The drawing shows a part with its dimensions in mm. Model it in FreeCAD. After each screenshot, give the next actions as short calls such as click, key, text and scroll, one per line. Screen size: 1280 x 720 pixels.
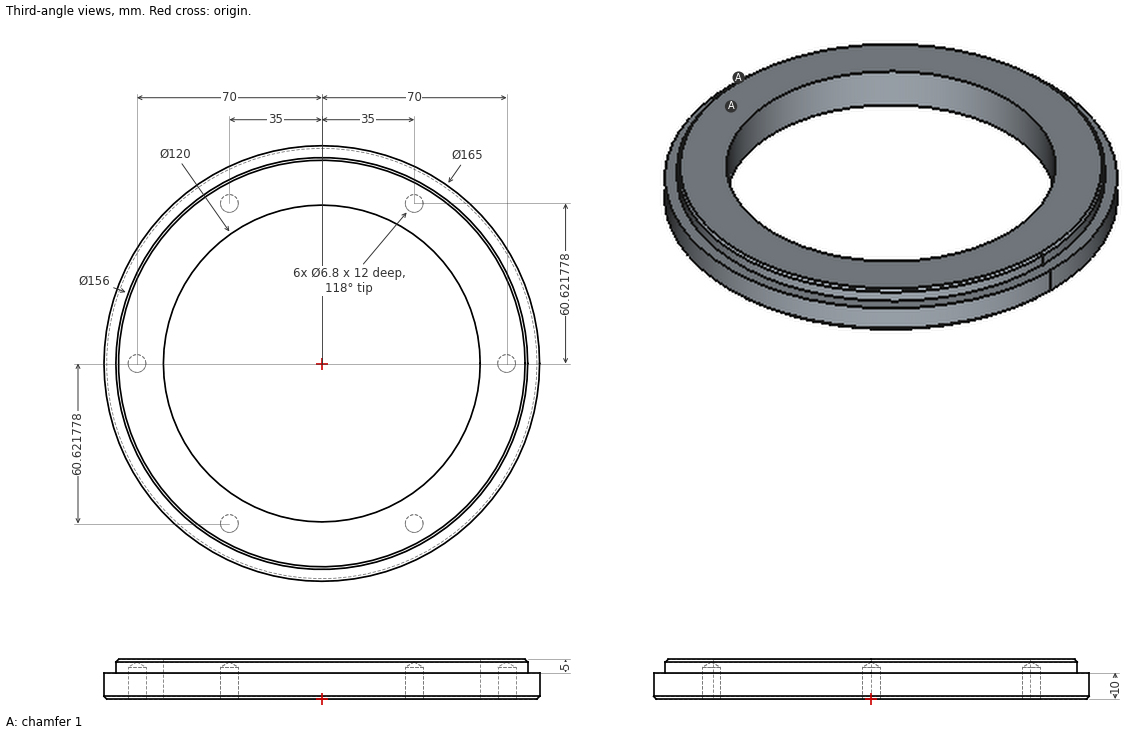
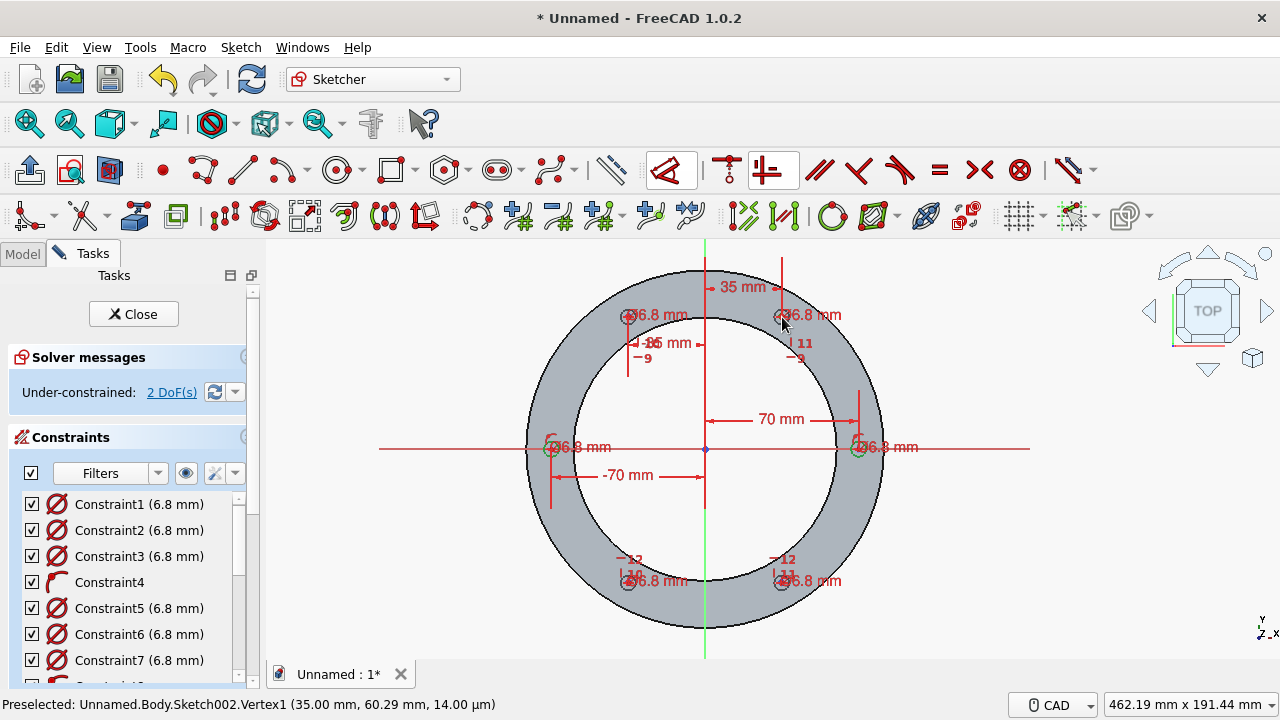
click(692, 170)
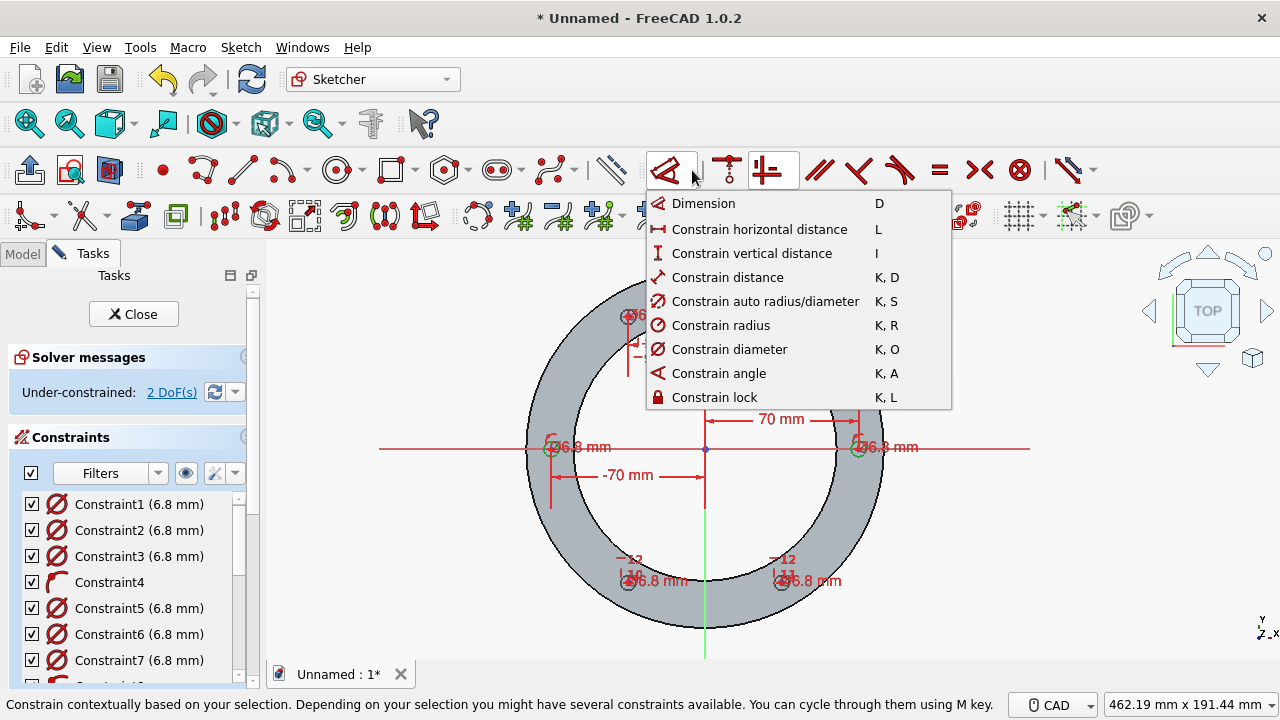
click(799, 253)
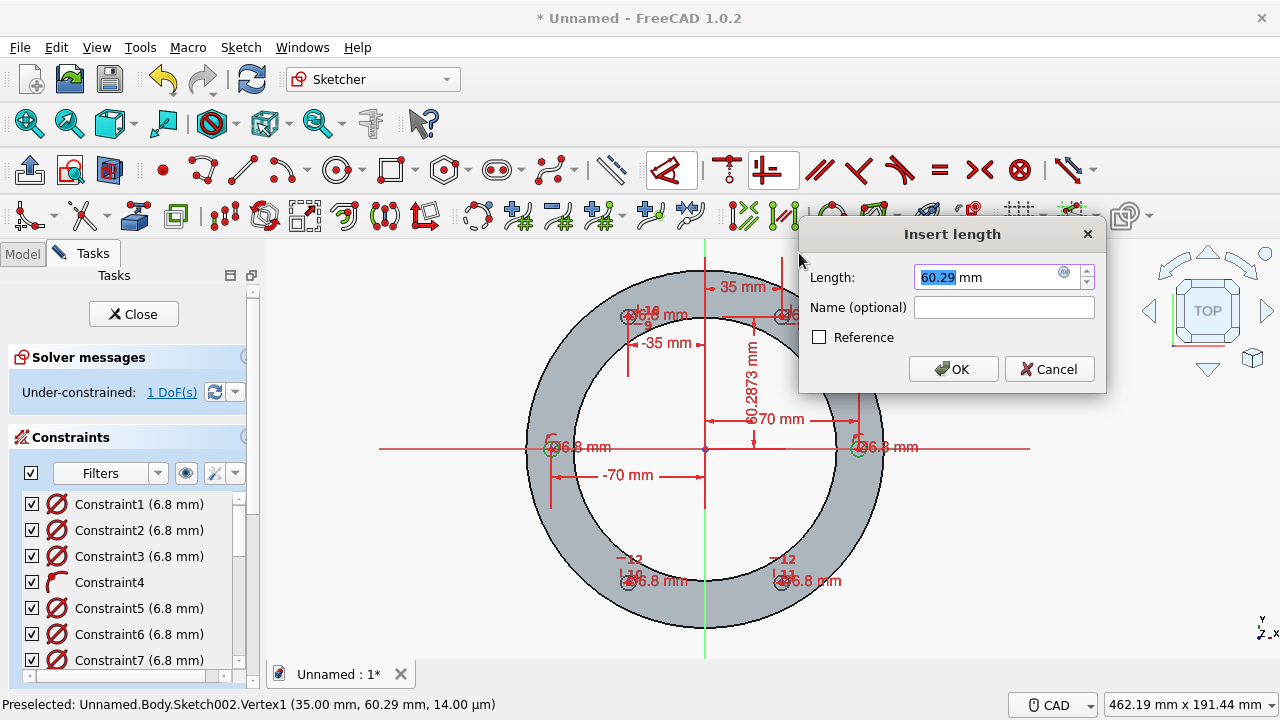
text(60.621778)
key(Return)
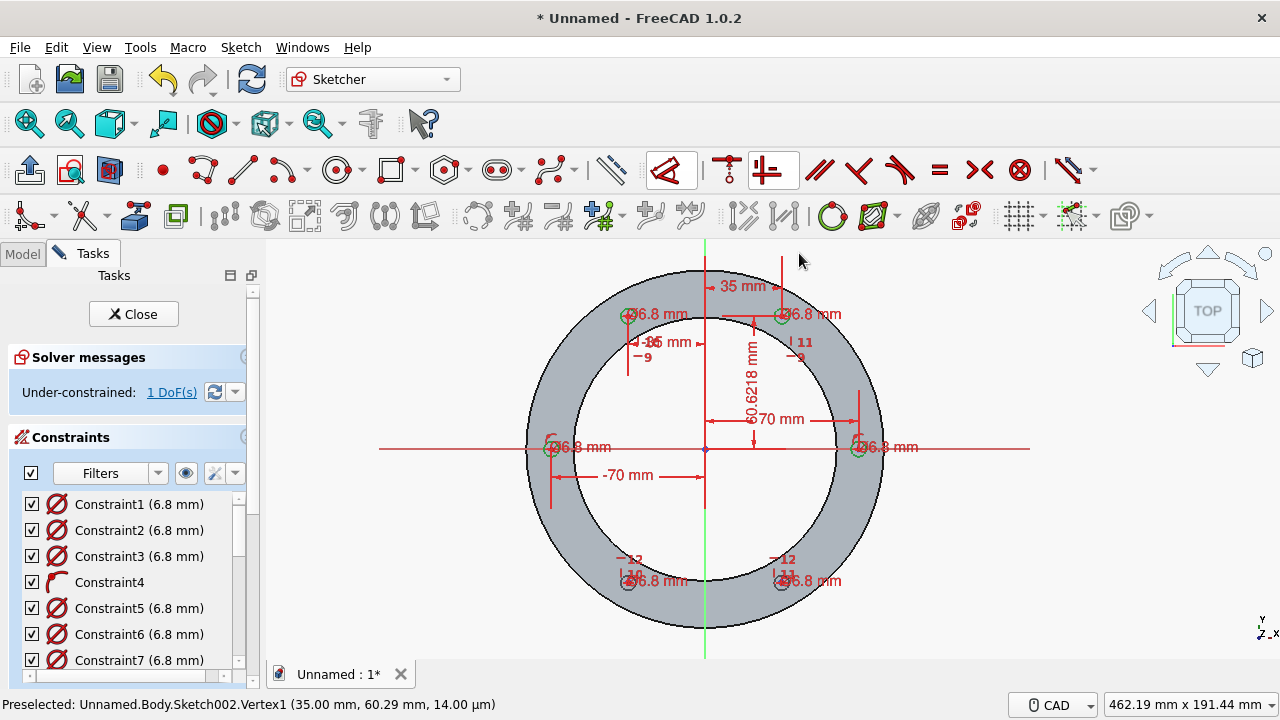
click(628, 583)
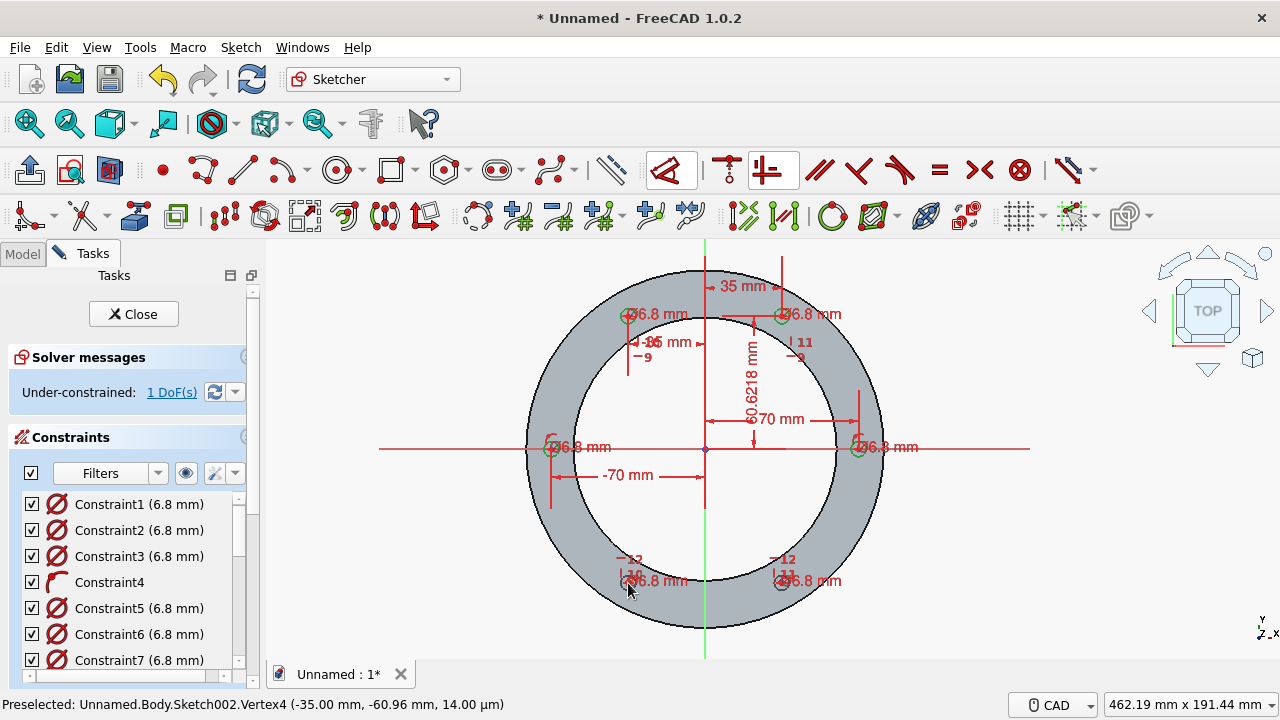
key(i)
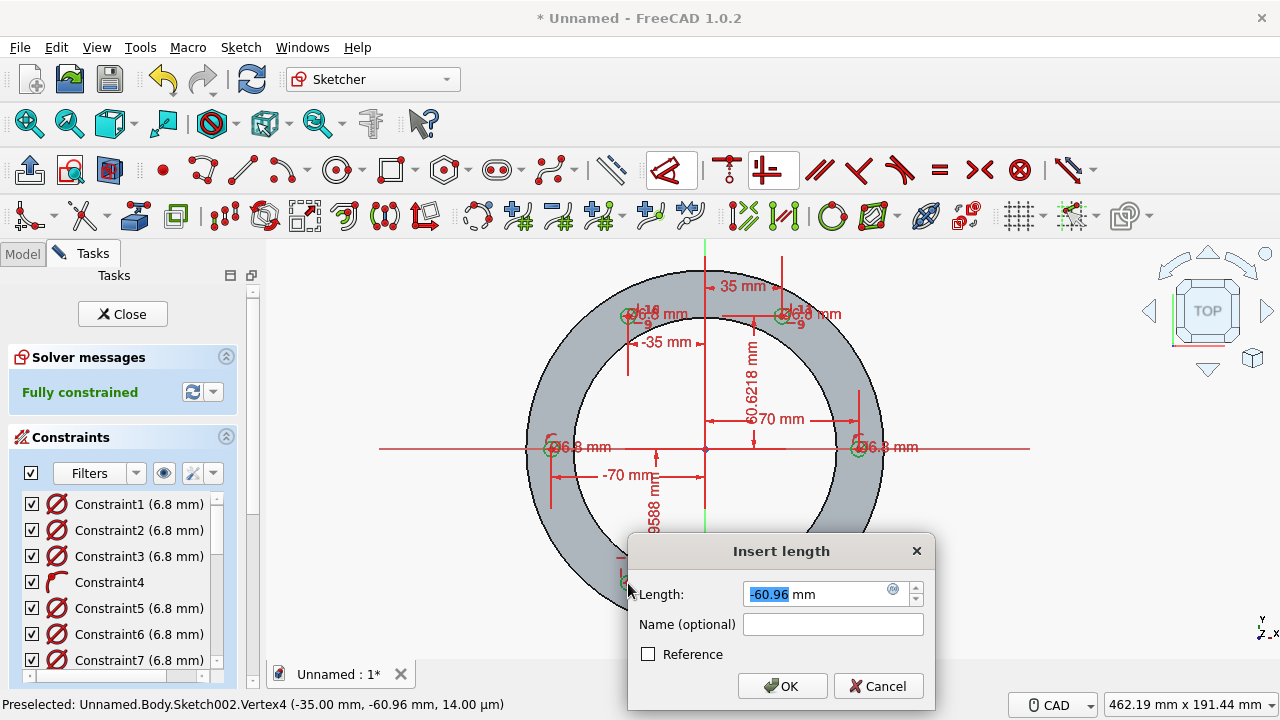
text(-60.621778)
key(Return)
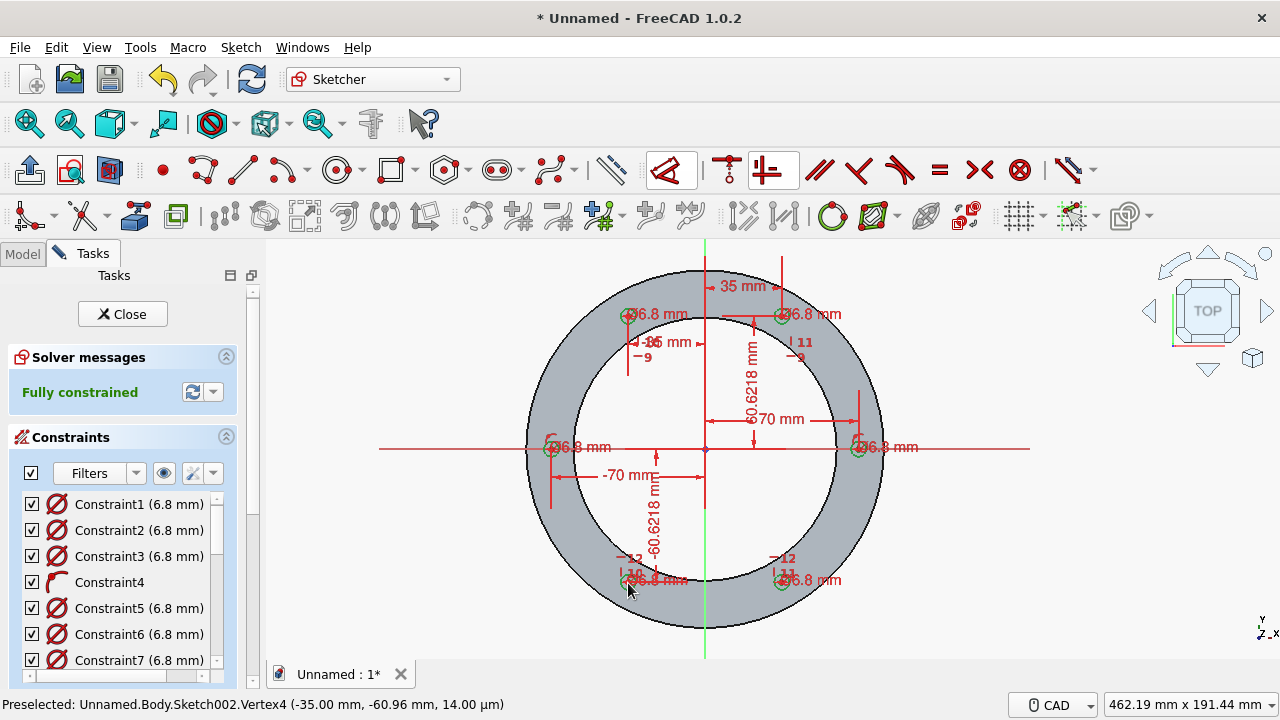
click(123, 314)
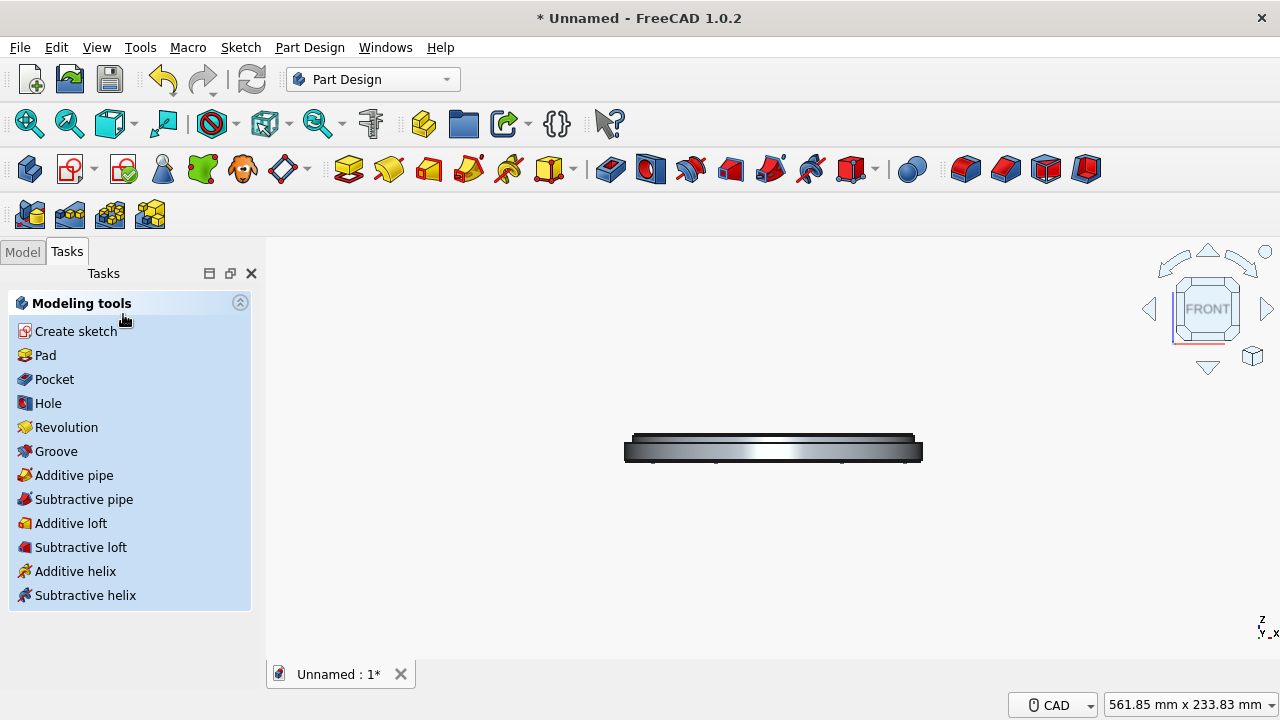
click(652, 170)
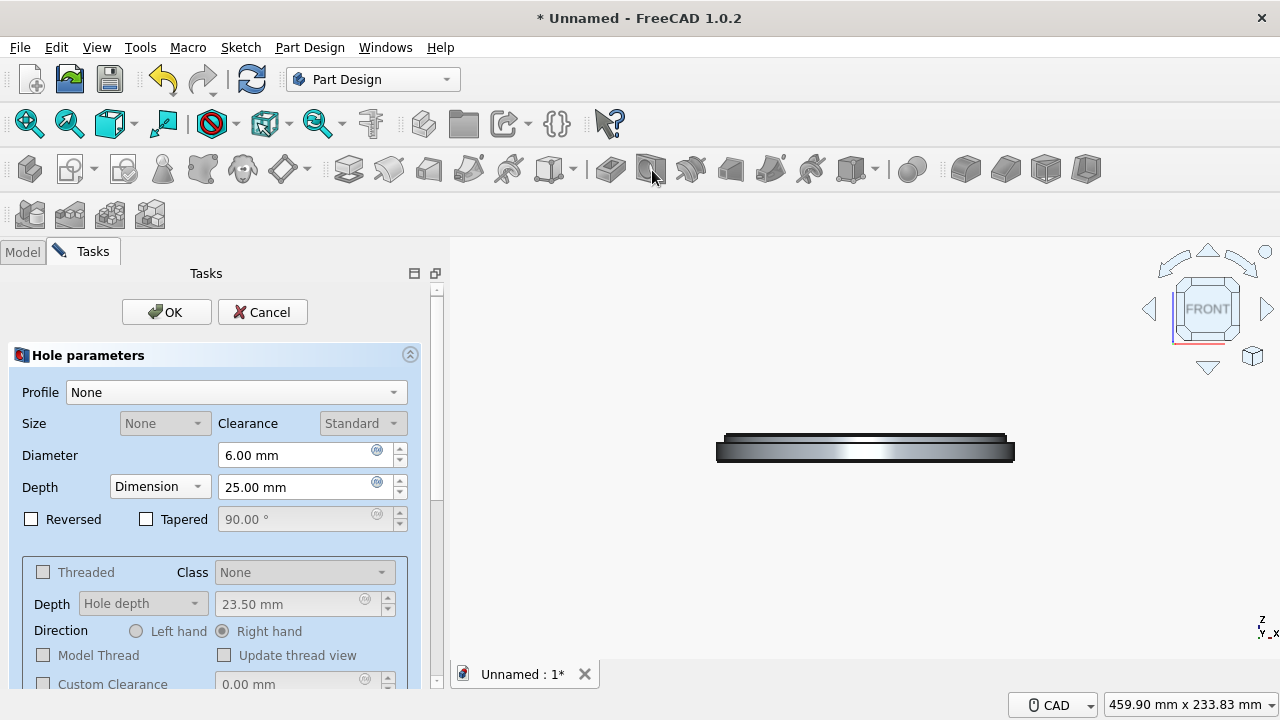
triple_click(305, 455)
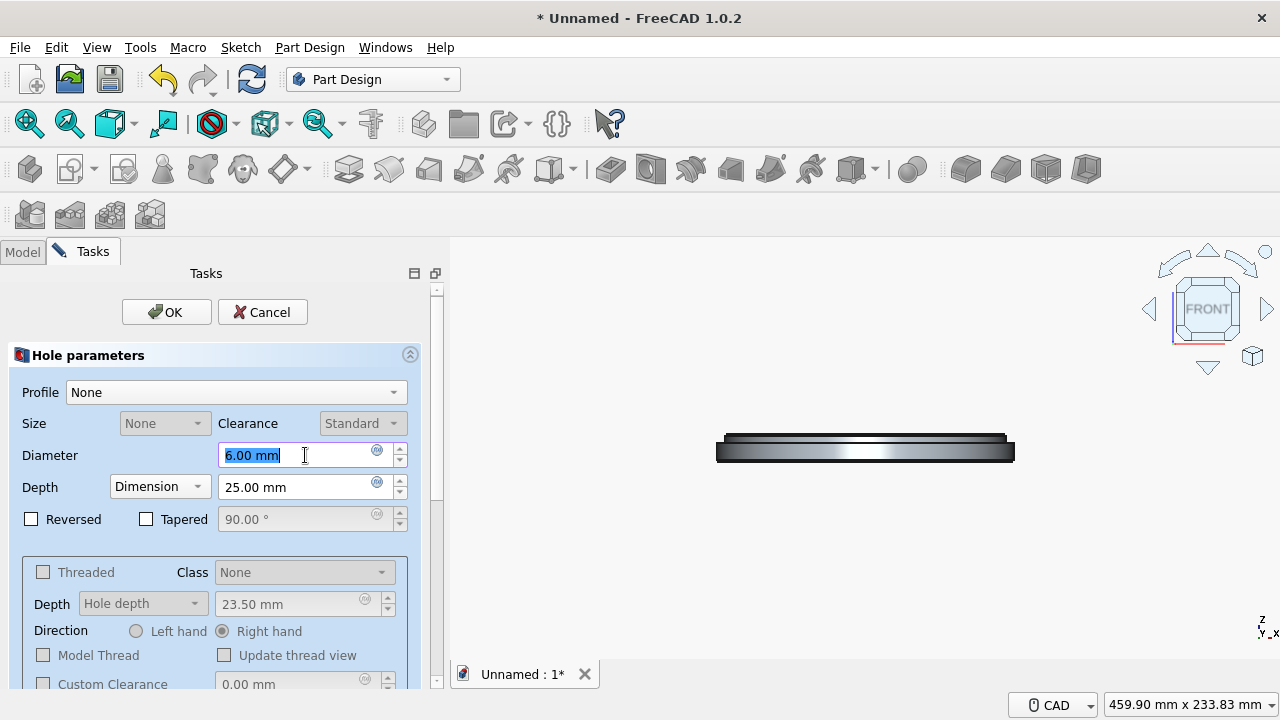
text(6.8)
key(Tab)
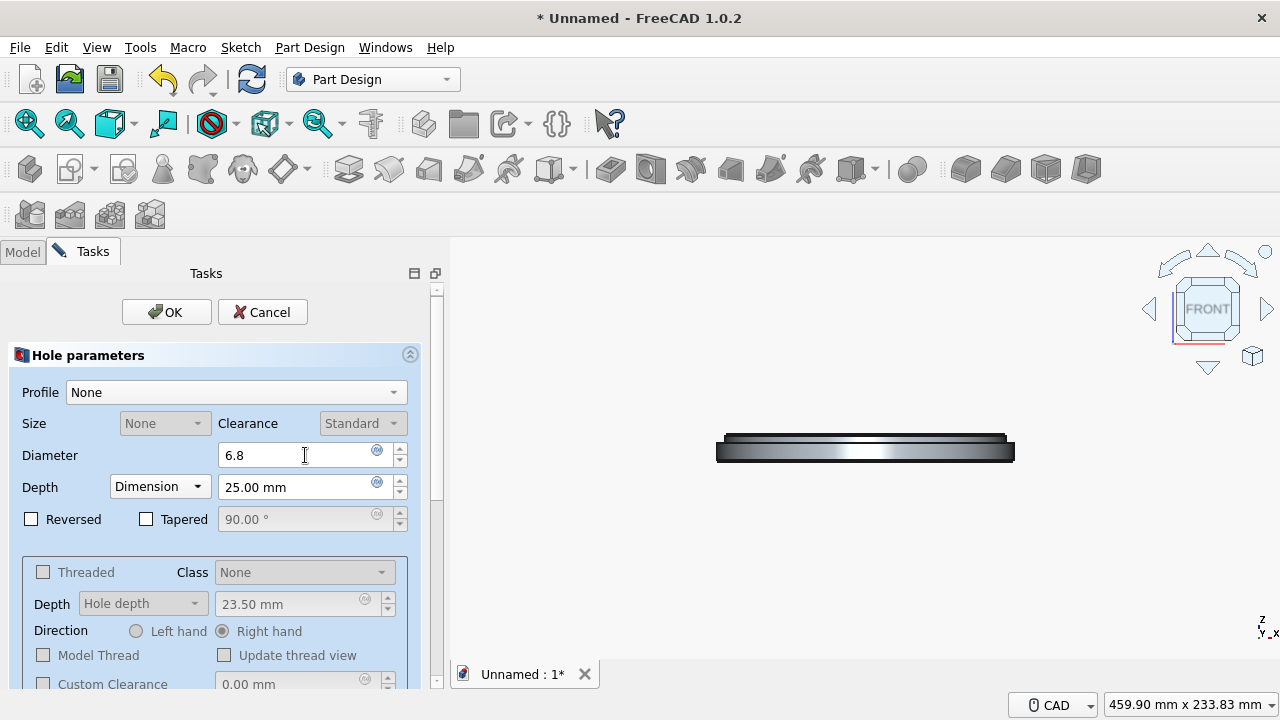
triple_click(305, 487)